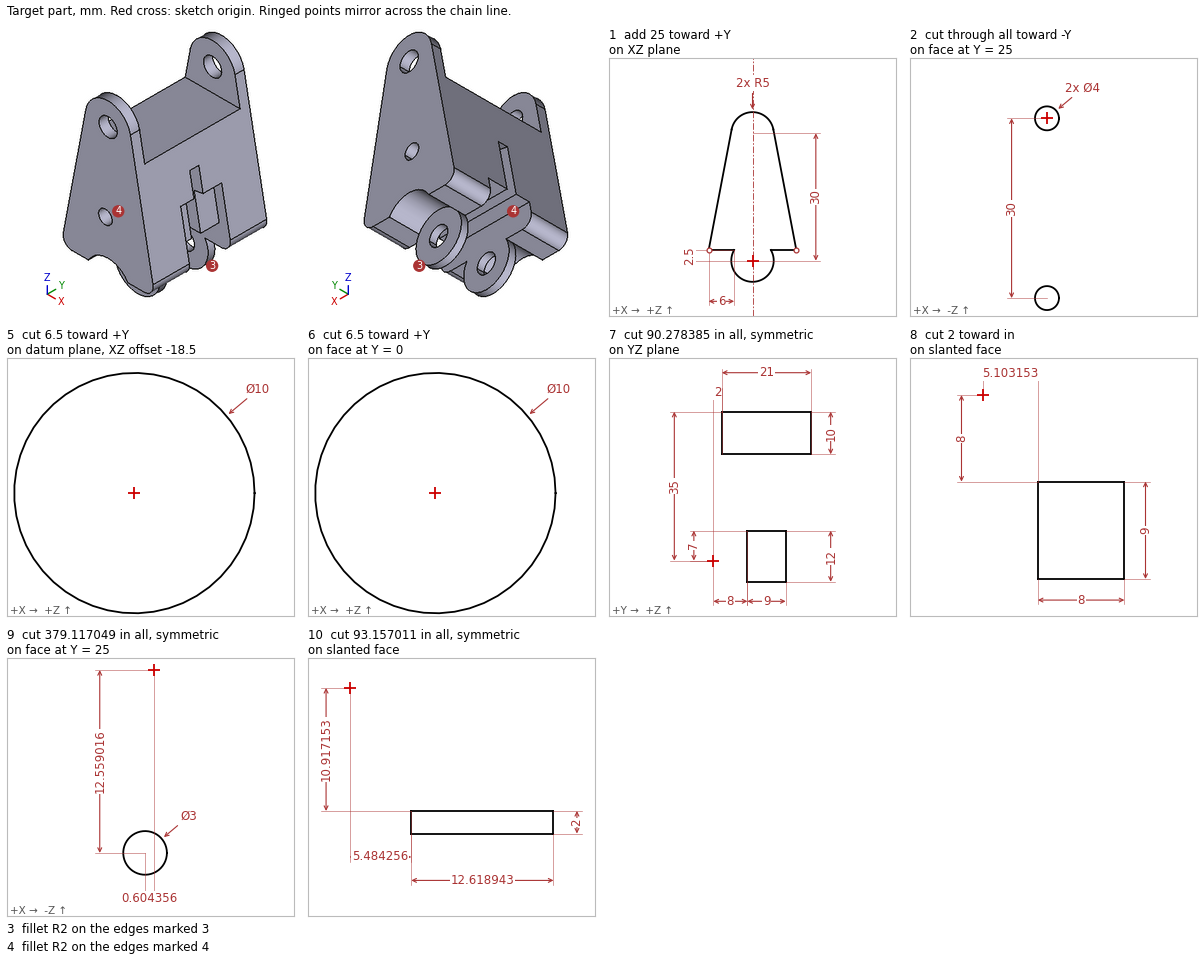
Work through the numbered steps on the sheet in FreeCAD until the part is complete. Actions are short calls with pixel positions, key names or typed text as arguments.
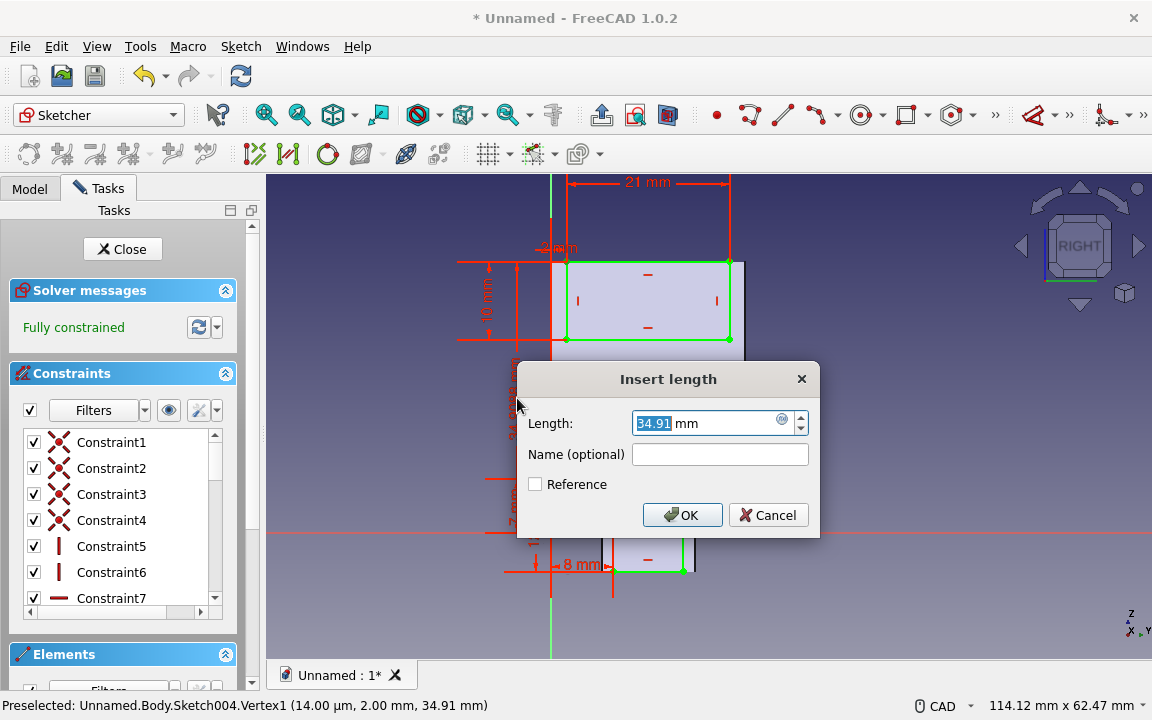
text(35)
key(Return)
key(Escape)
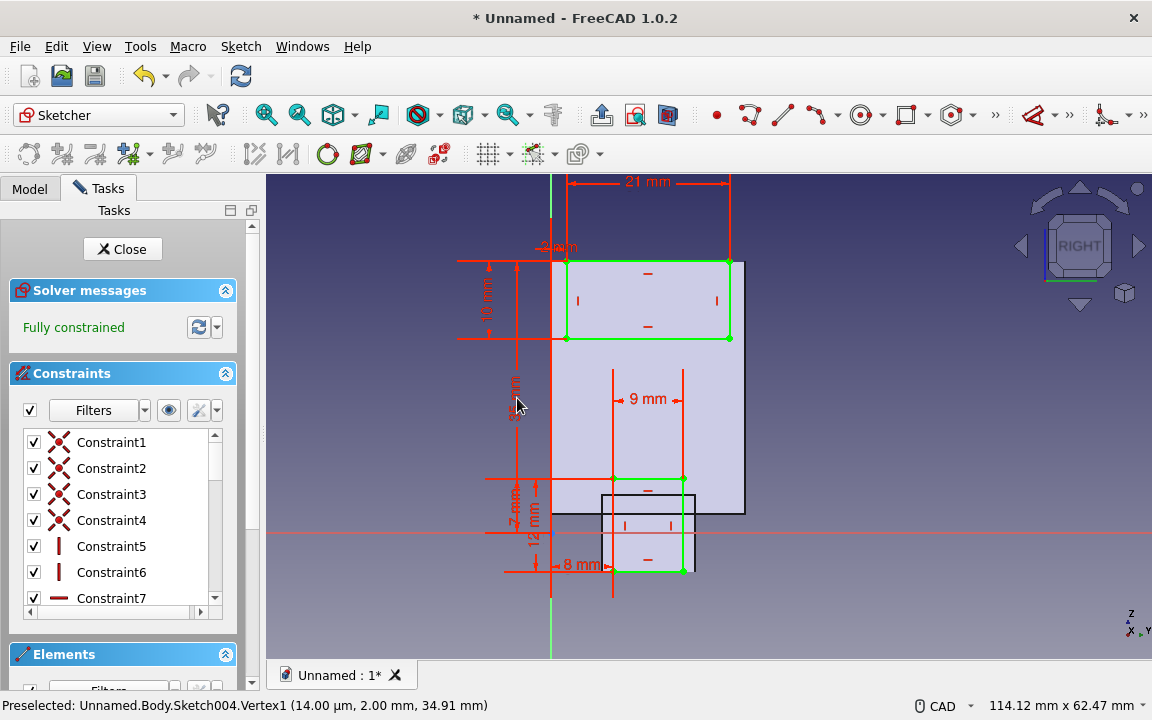
click(123, 249)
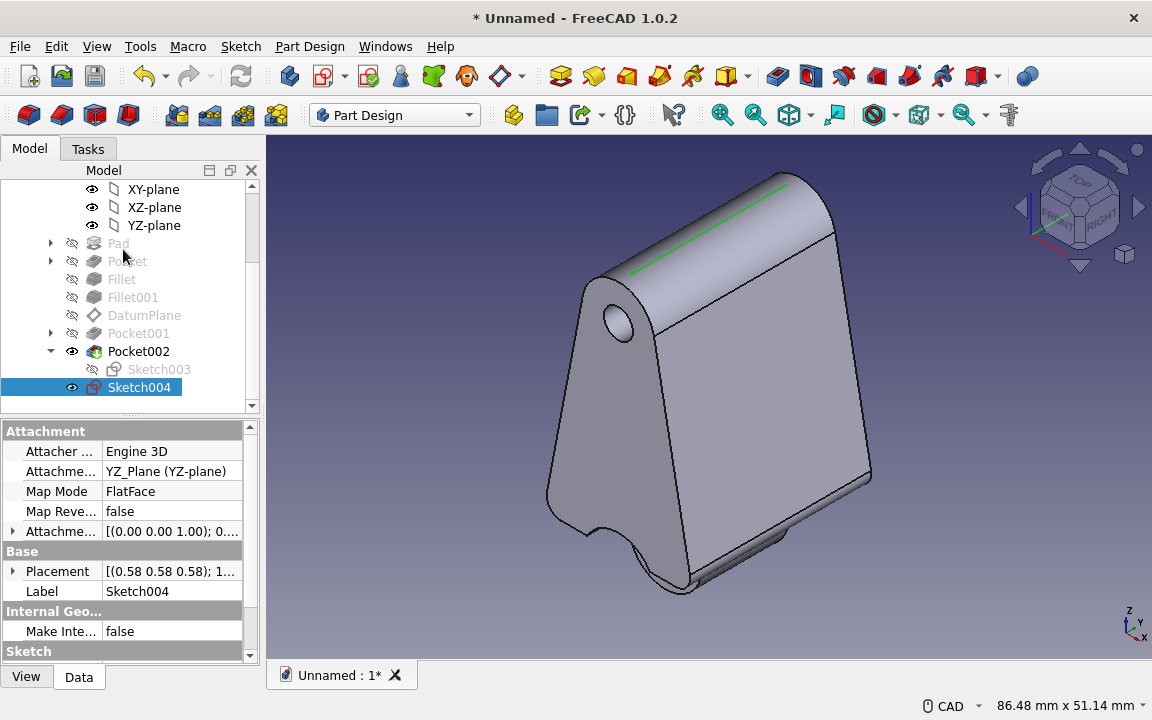
click(778, 76)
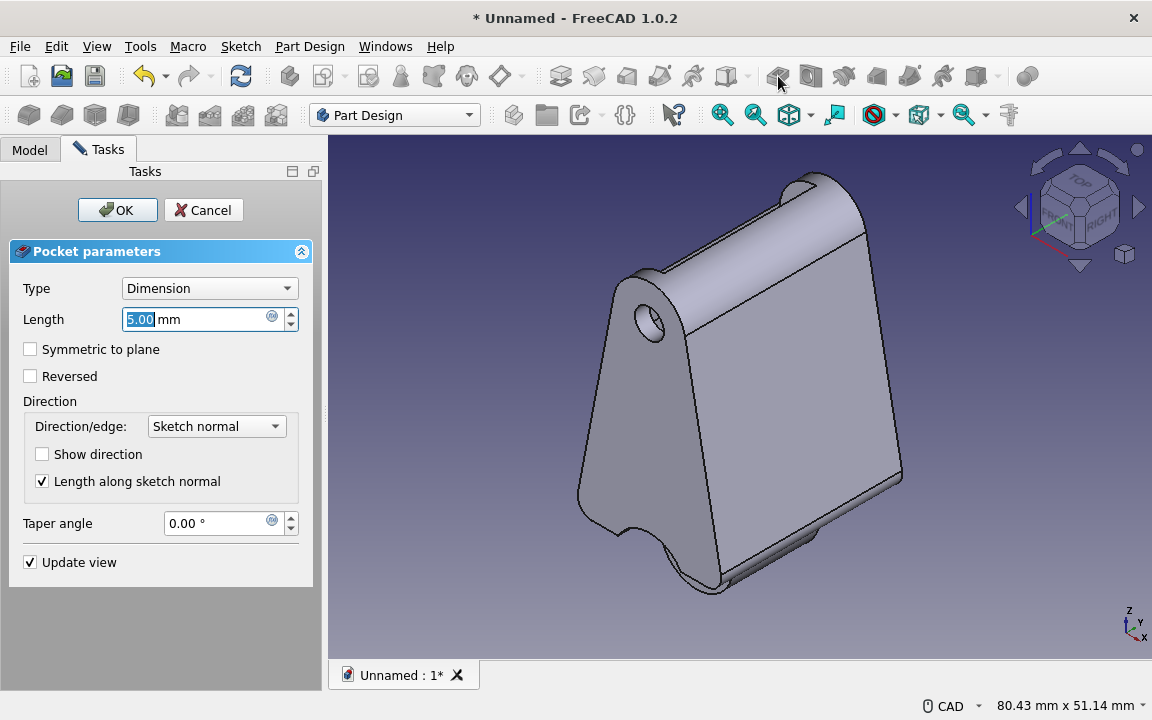
text(90.278385)
key(Tab)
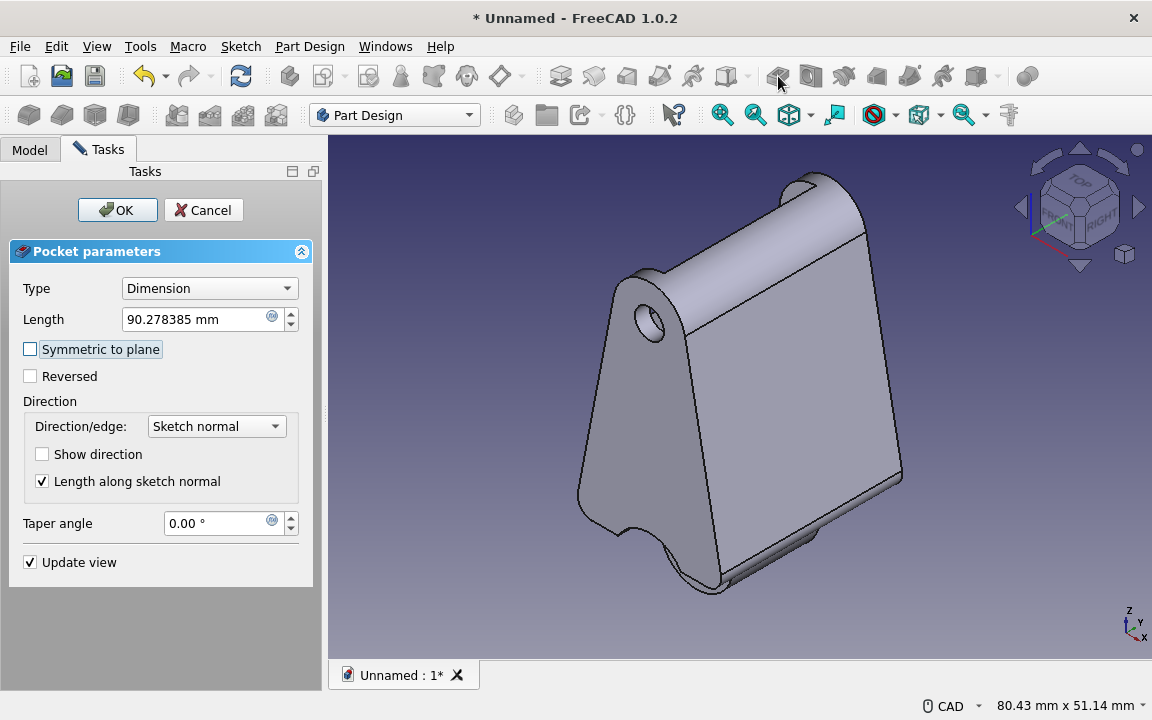
click(31, 349)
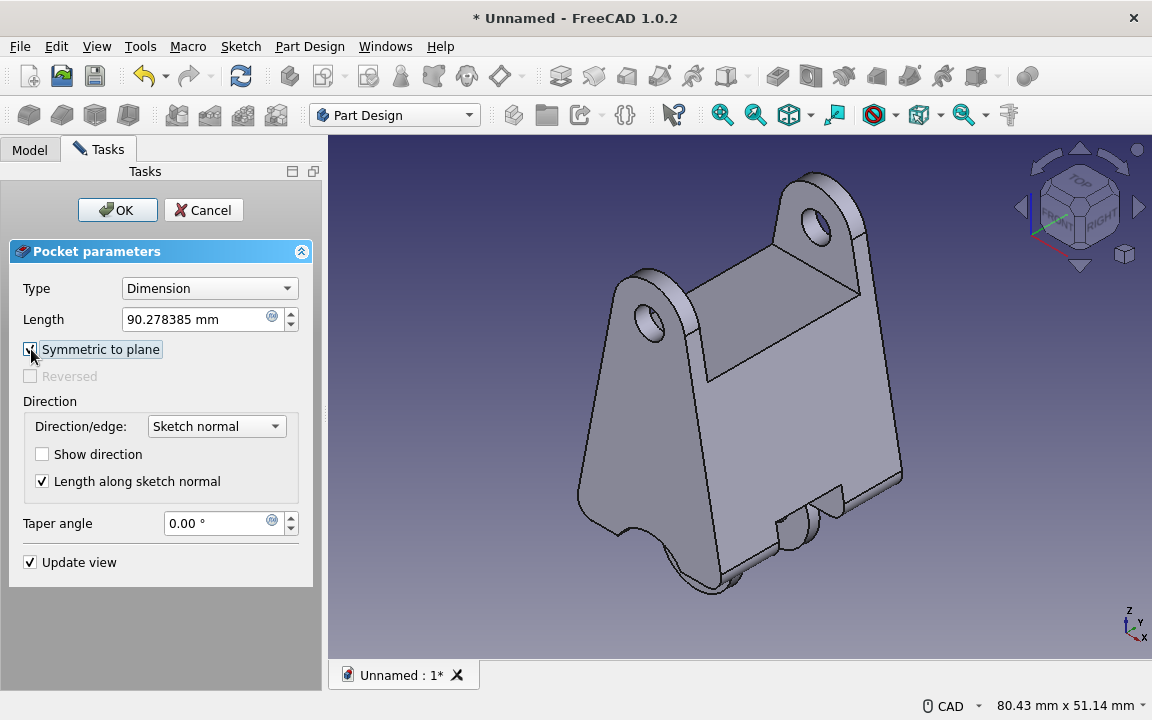
click(118, 210)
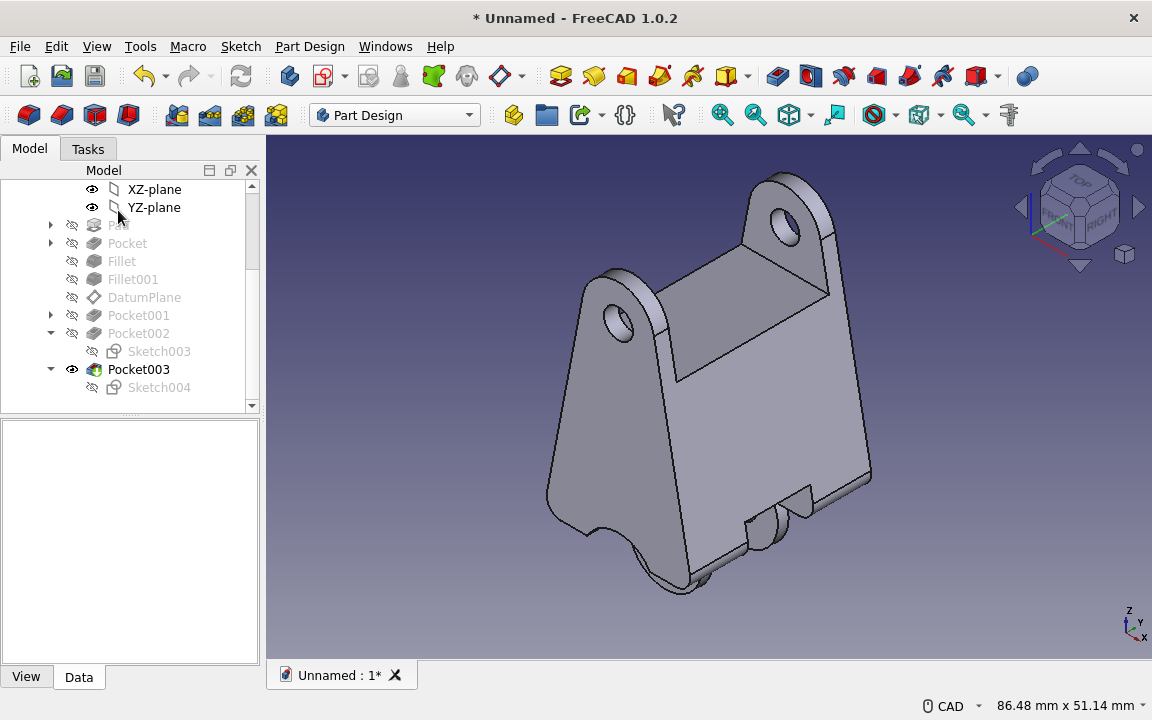
click(742, 452)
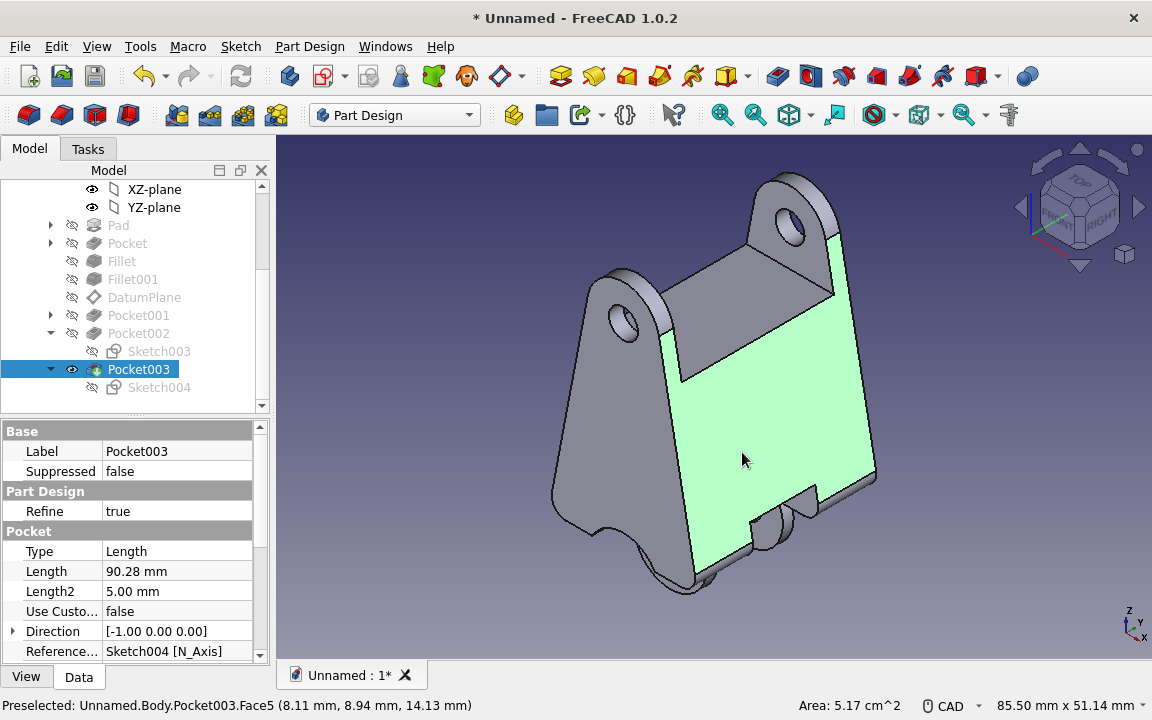
click(322, 76)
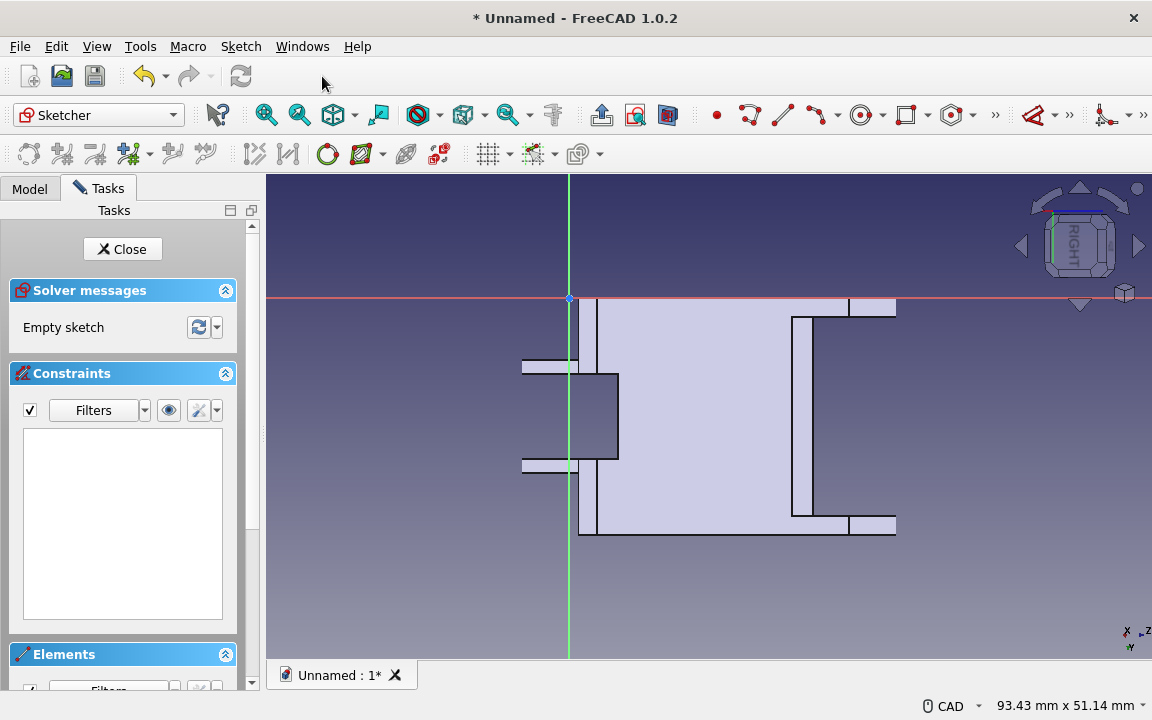
scroll(621, 333, up, 3)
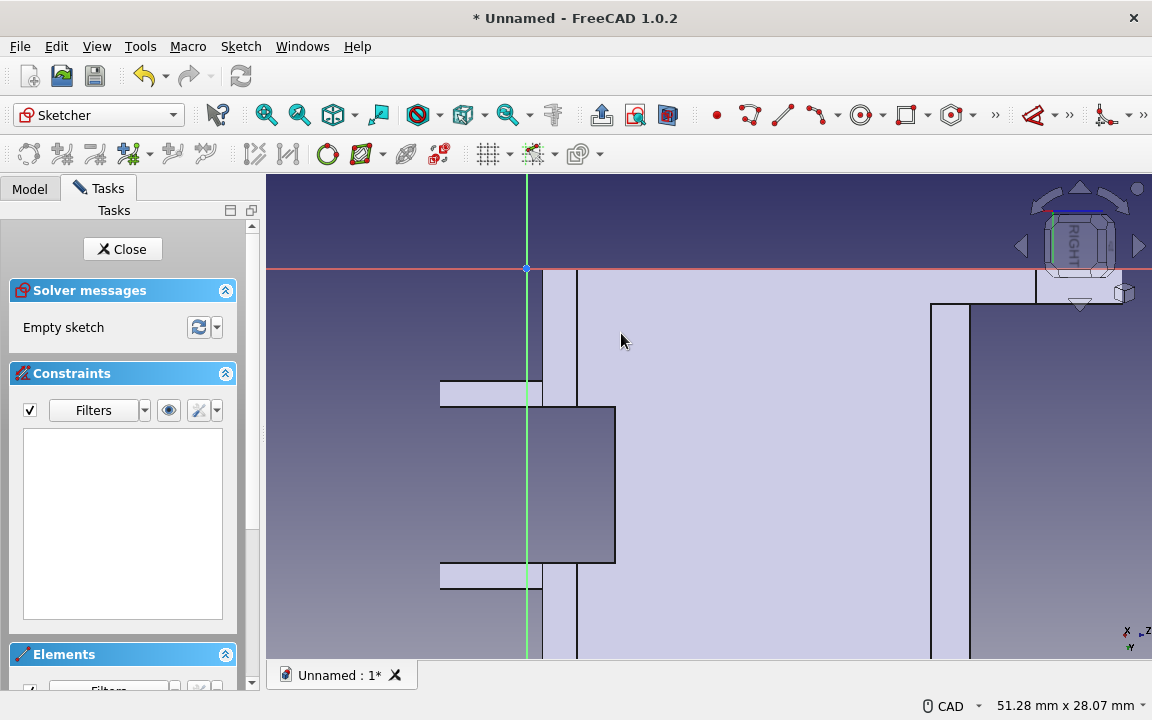
key(g)
key(r)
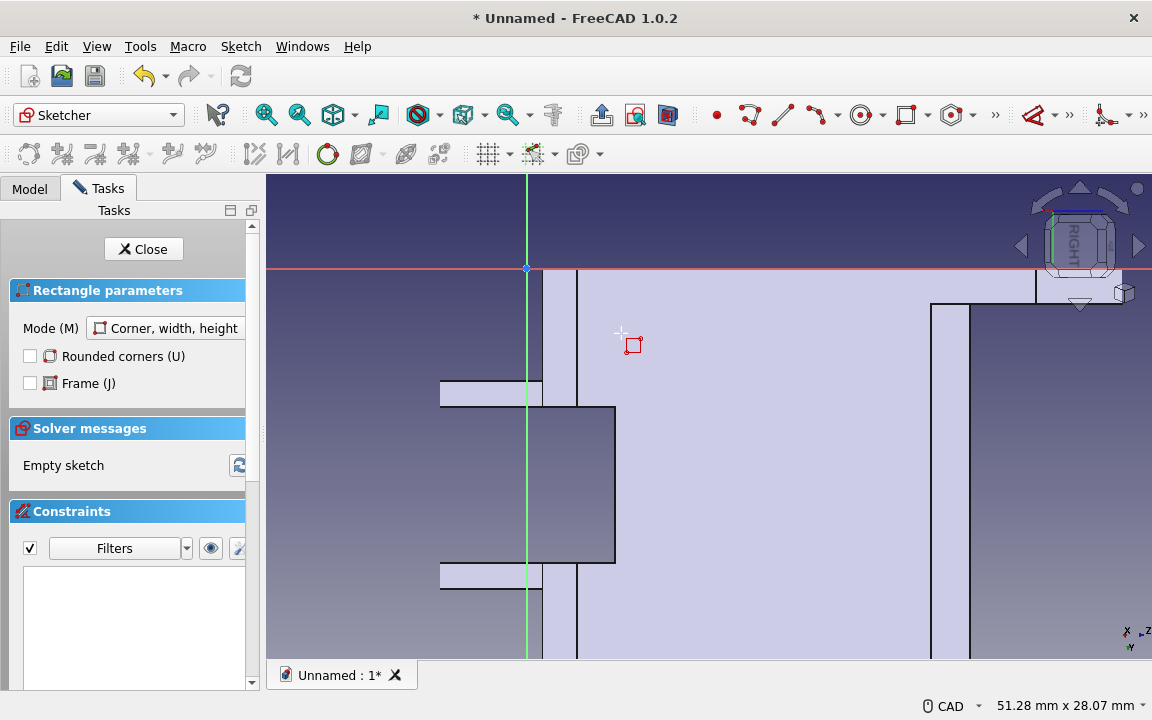
click(615, 407)
move(753, 563)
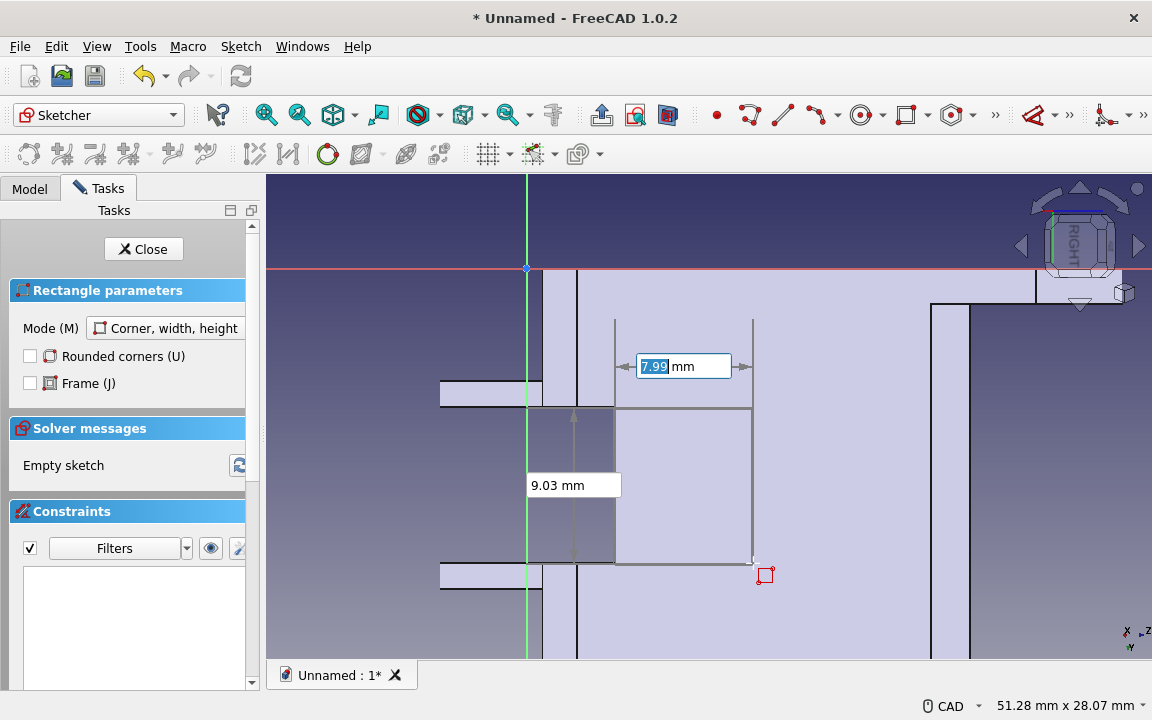
text(8)
key(Tab)
text(9)
key(Return)
key(Escape)